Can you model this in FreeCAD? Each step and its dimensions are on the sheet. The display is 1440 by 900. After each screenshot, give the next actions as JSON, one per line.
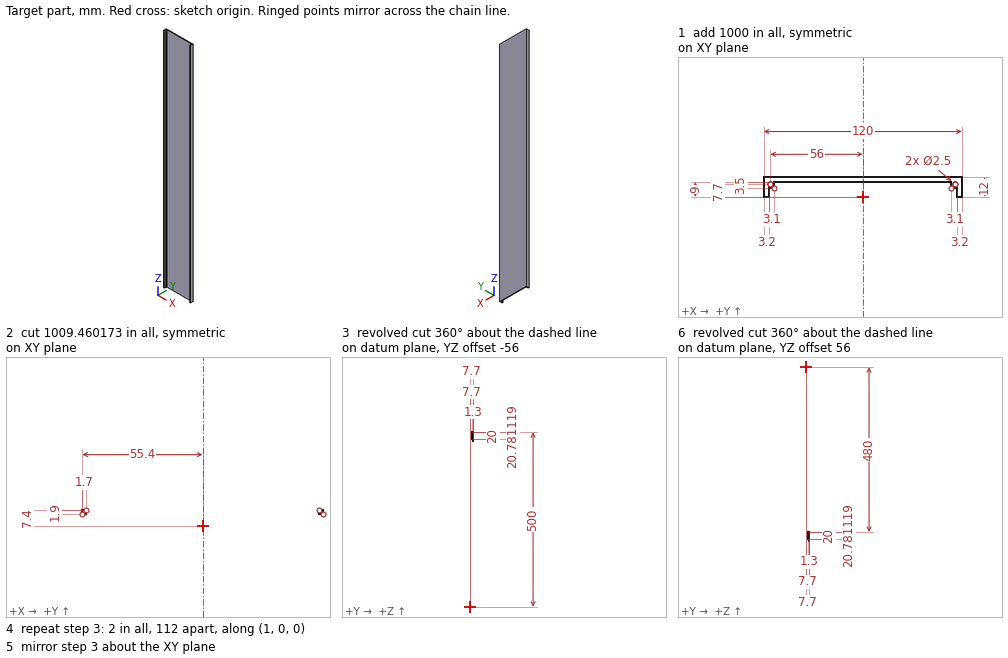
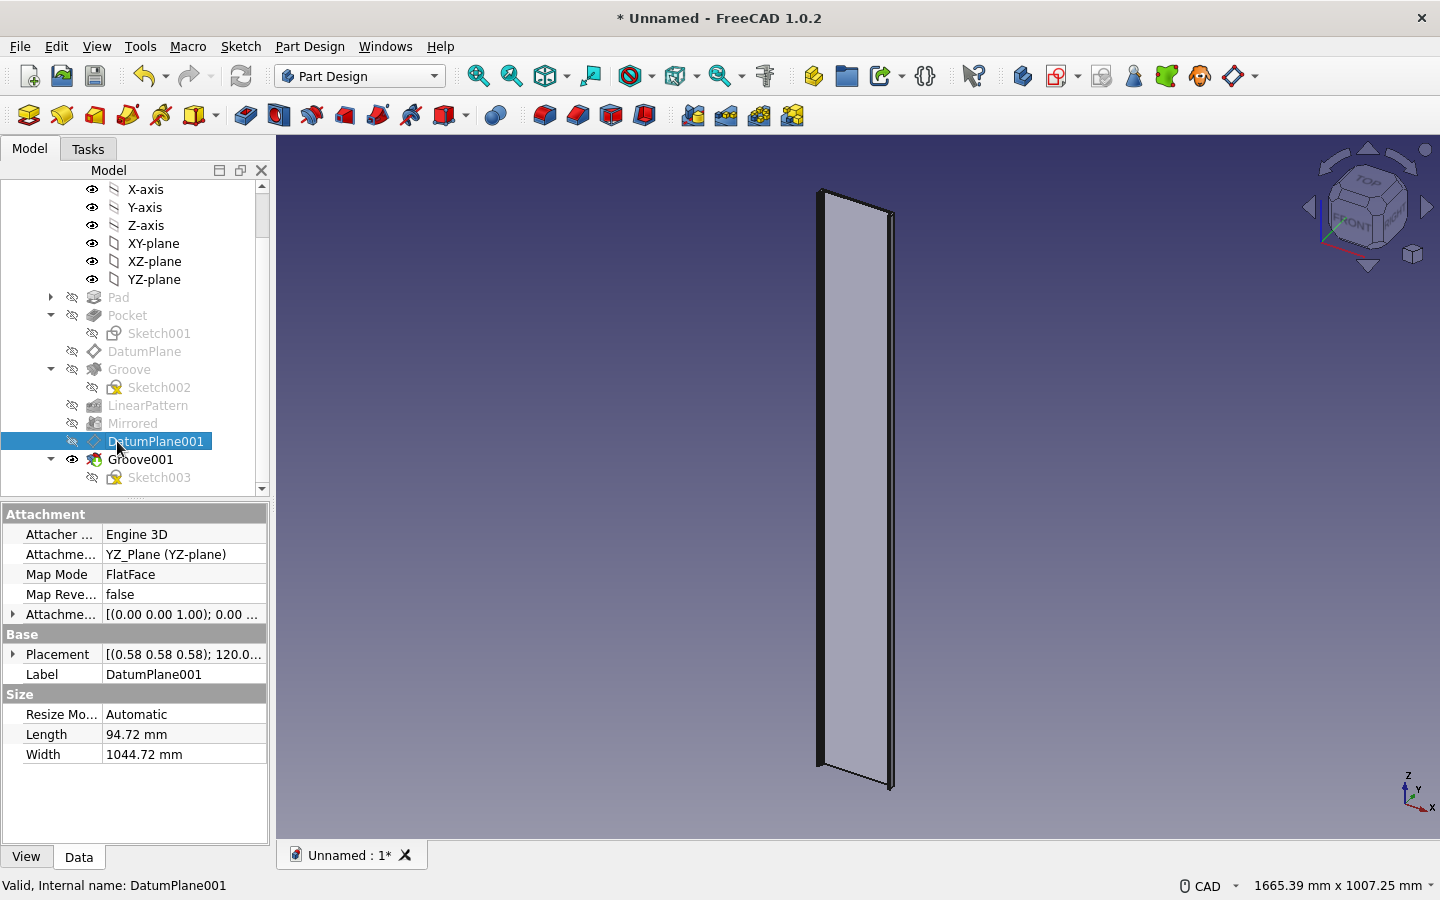
{"action": "key", "text": "0"}